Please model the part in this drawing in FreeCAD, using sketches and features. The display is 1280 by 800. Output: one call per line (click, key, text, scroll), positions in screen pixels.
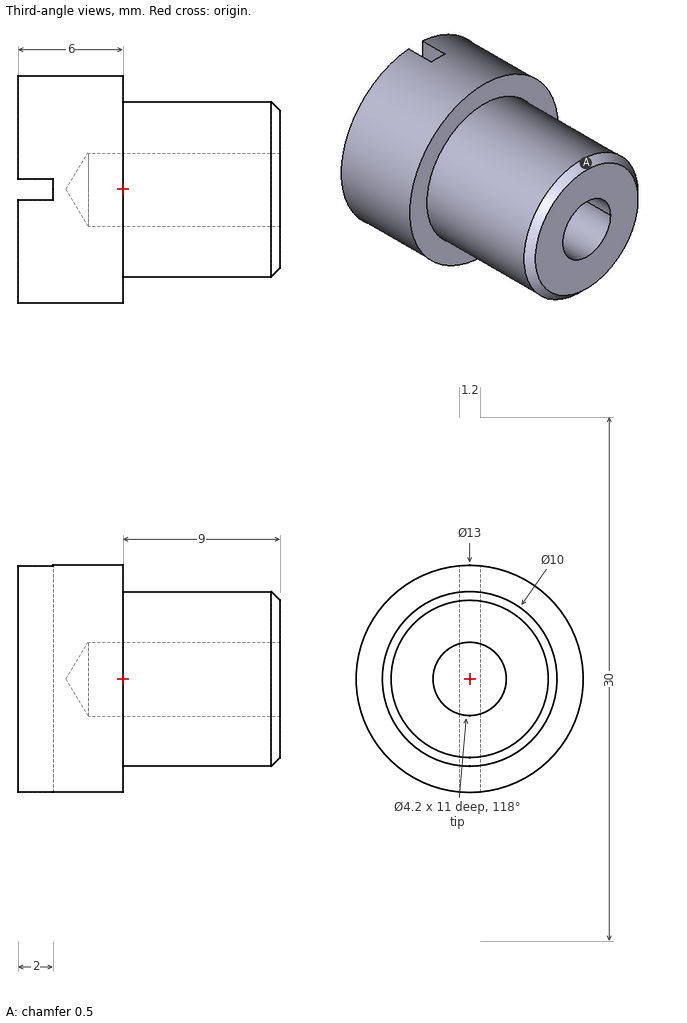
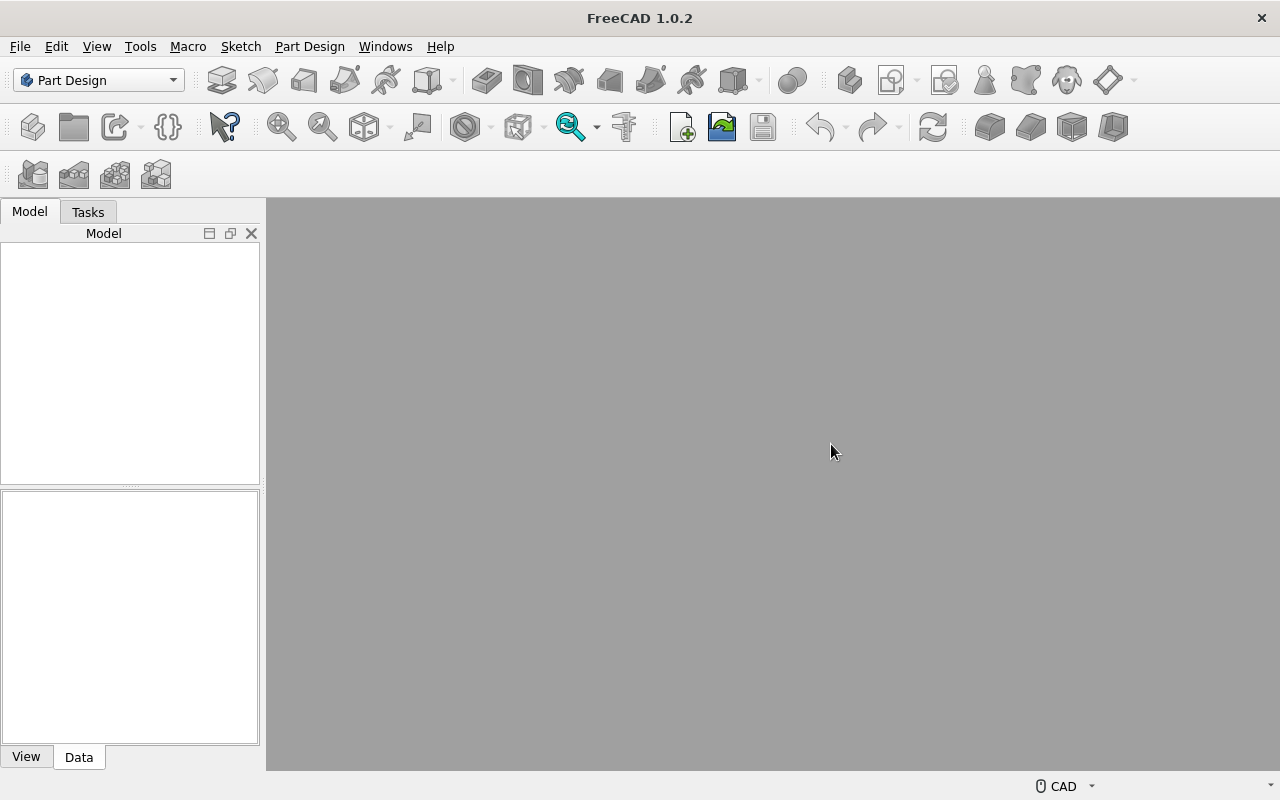
click(681, 128)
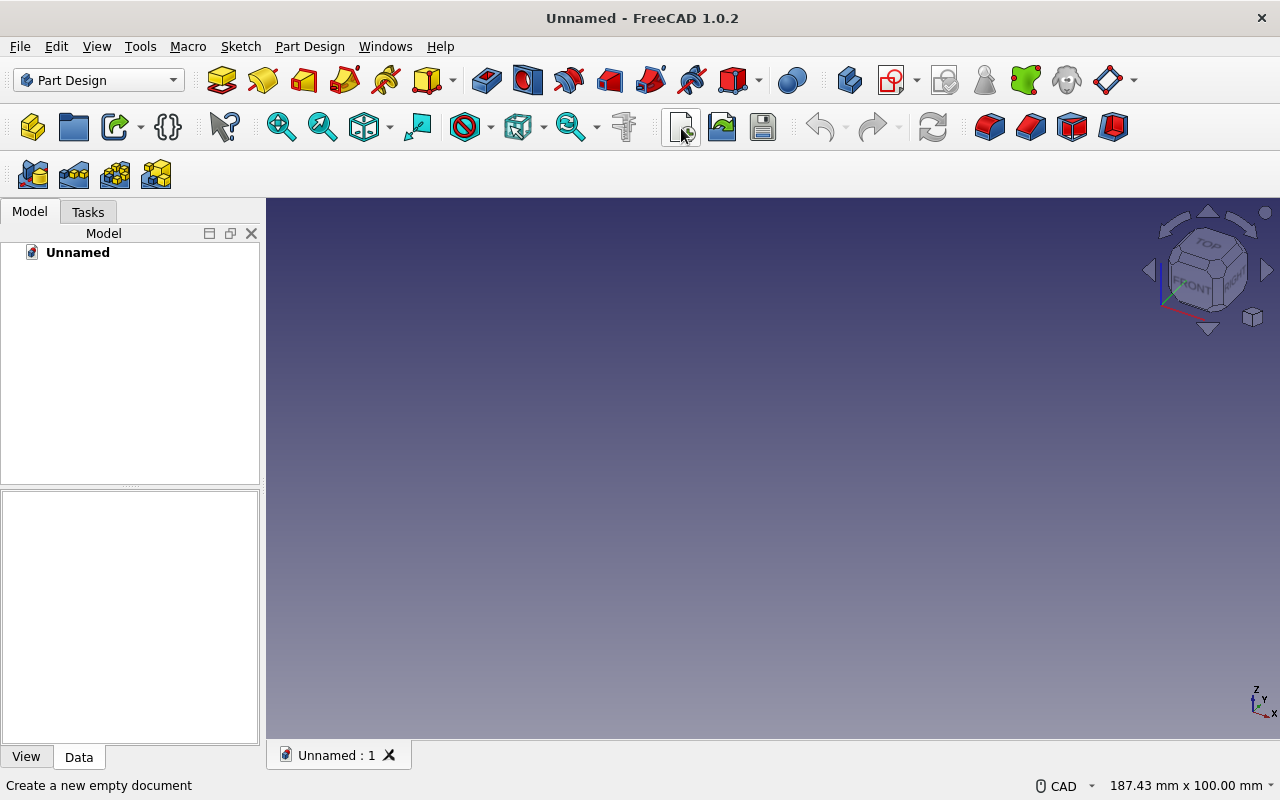
click(890, 80)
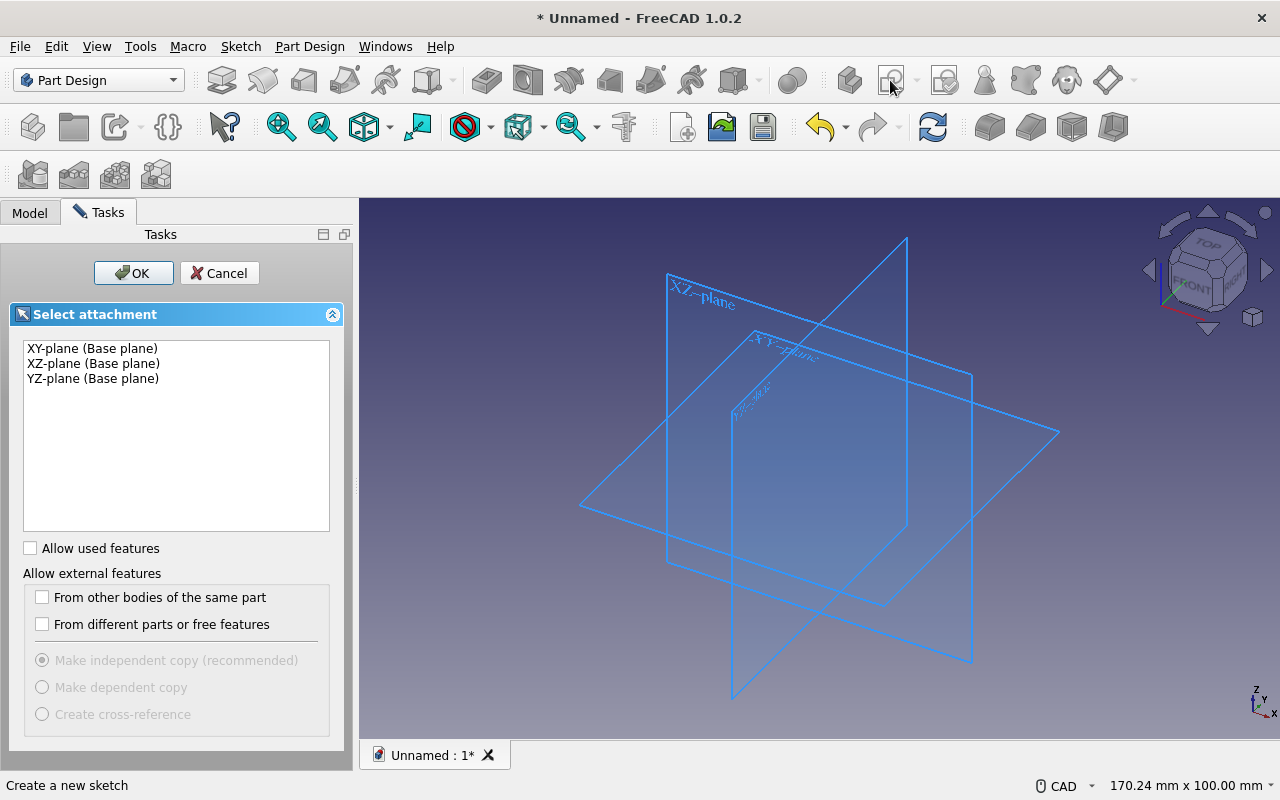
click(84, 378)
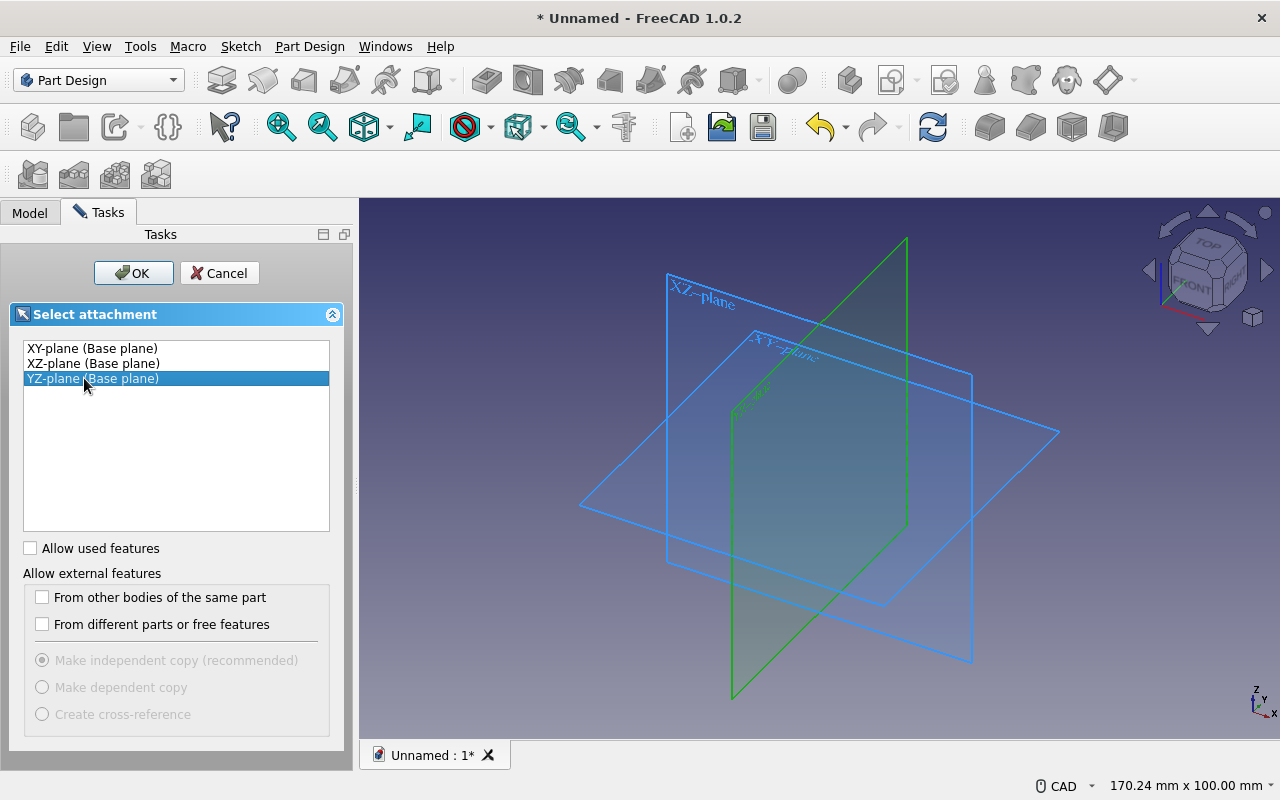
click(134, 273)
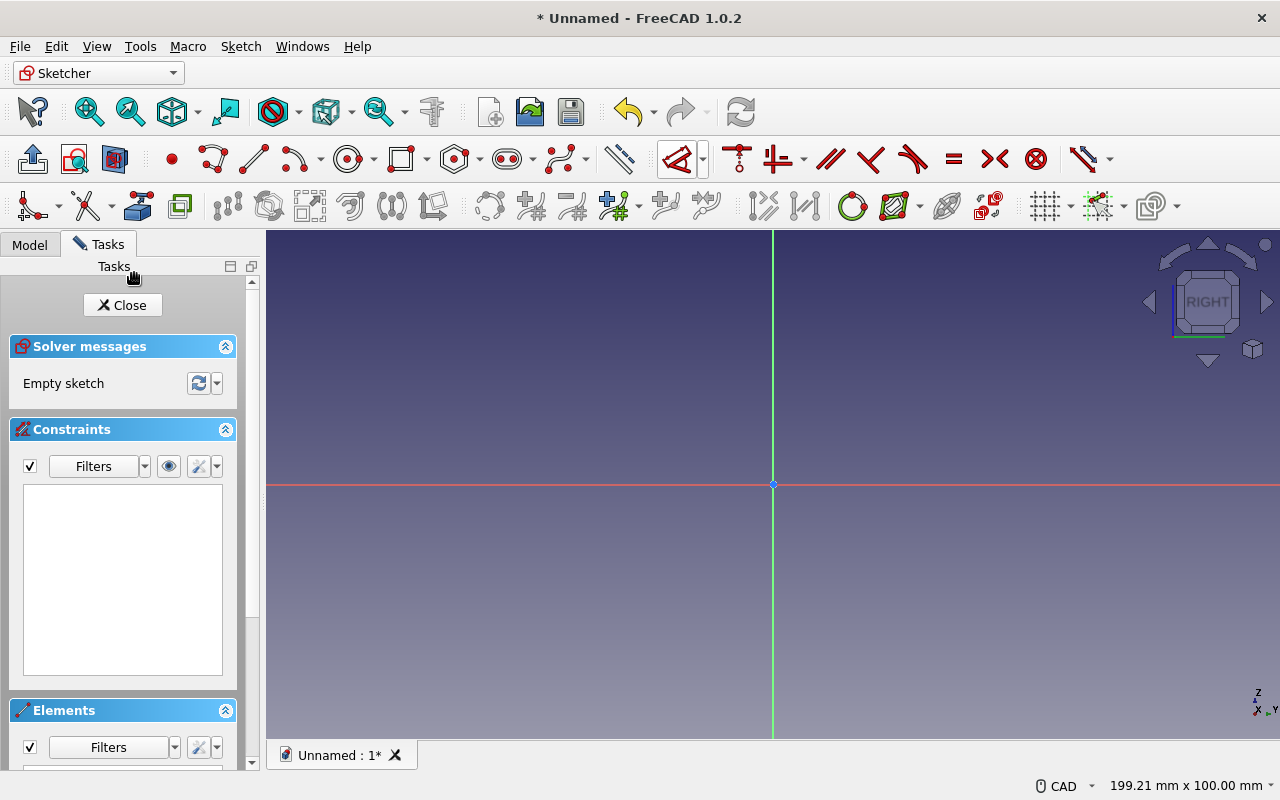
scroll(787, 484, up, 9)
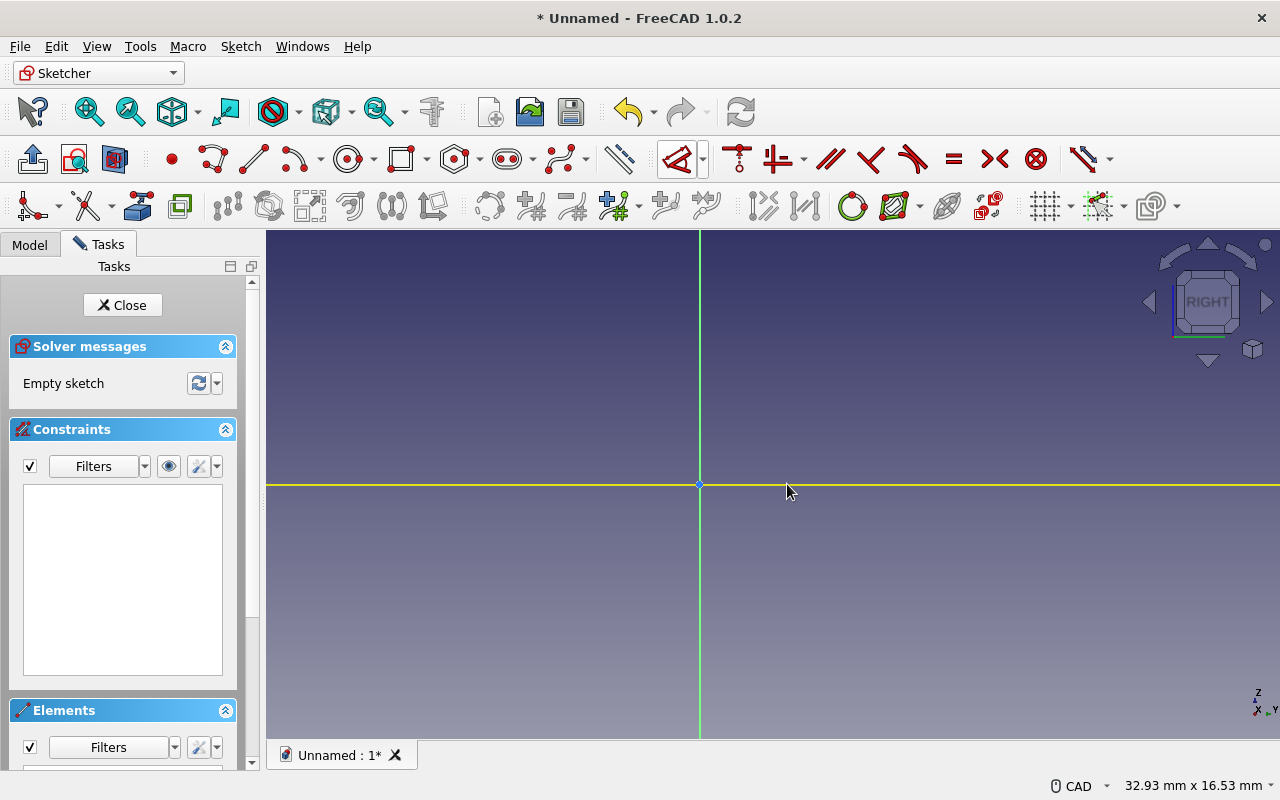
click(348, 160)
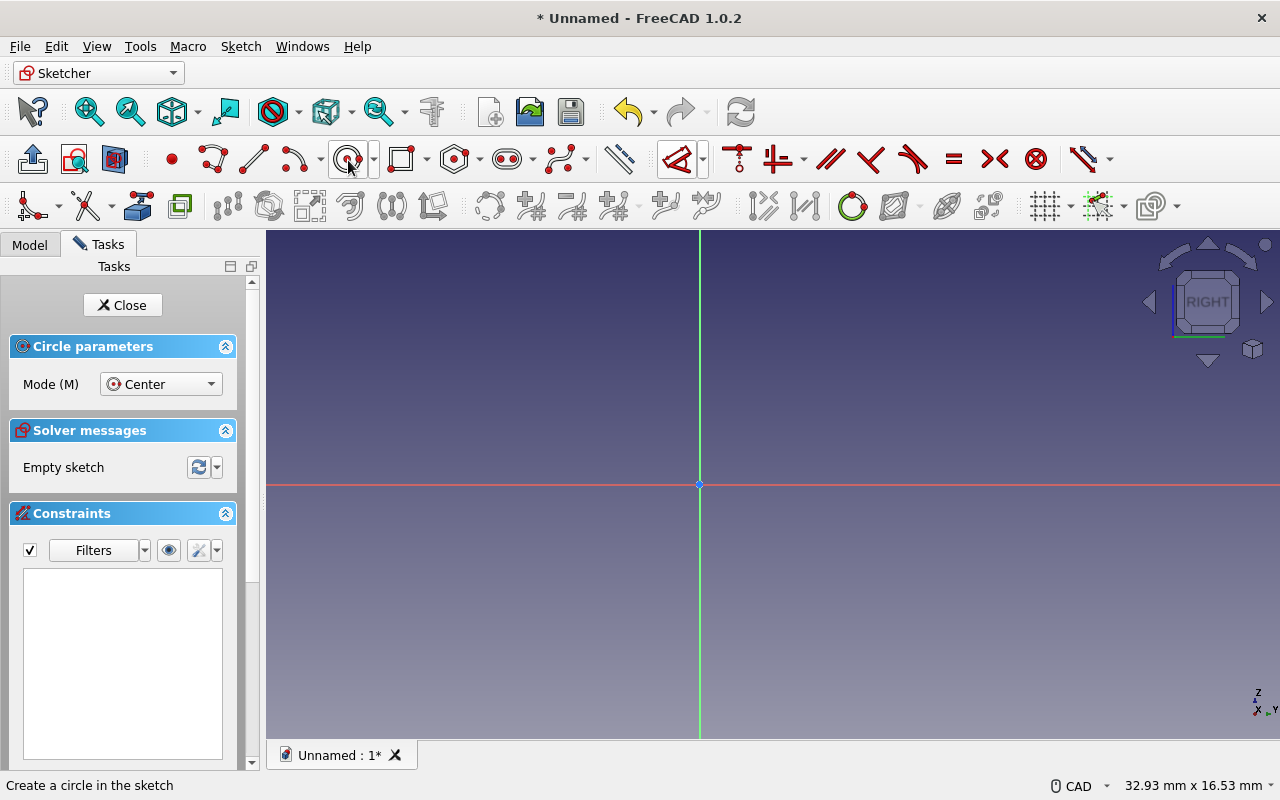
click(700, 484)
move(809, 376)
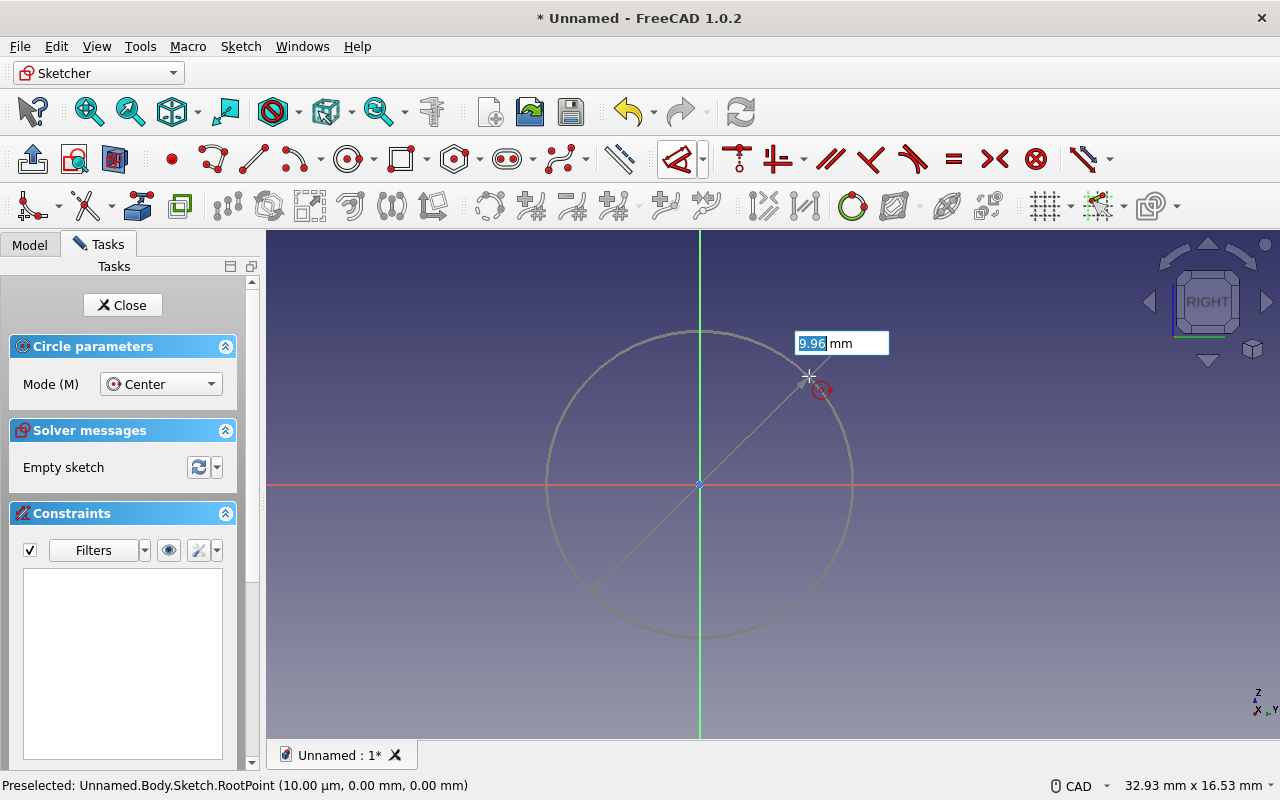
text(10)
key(Return)
key(Escape)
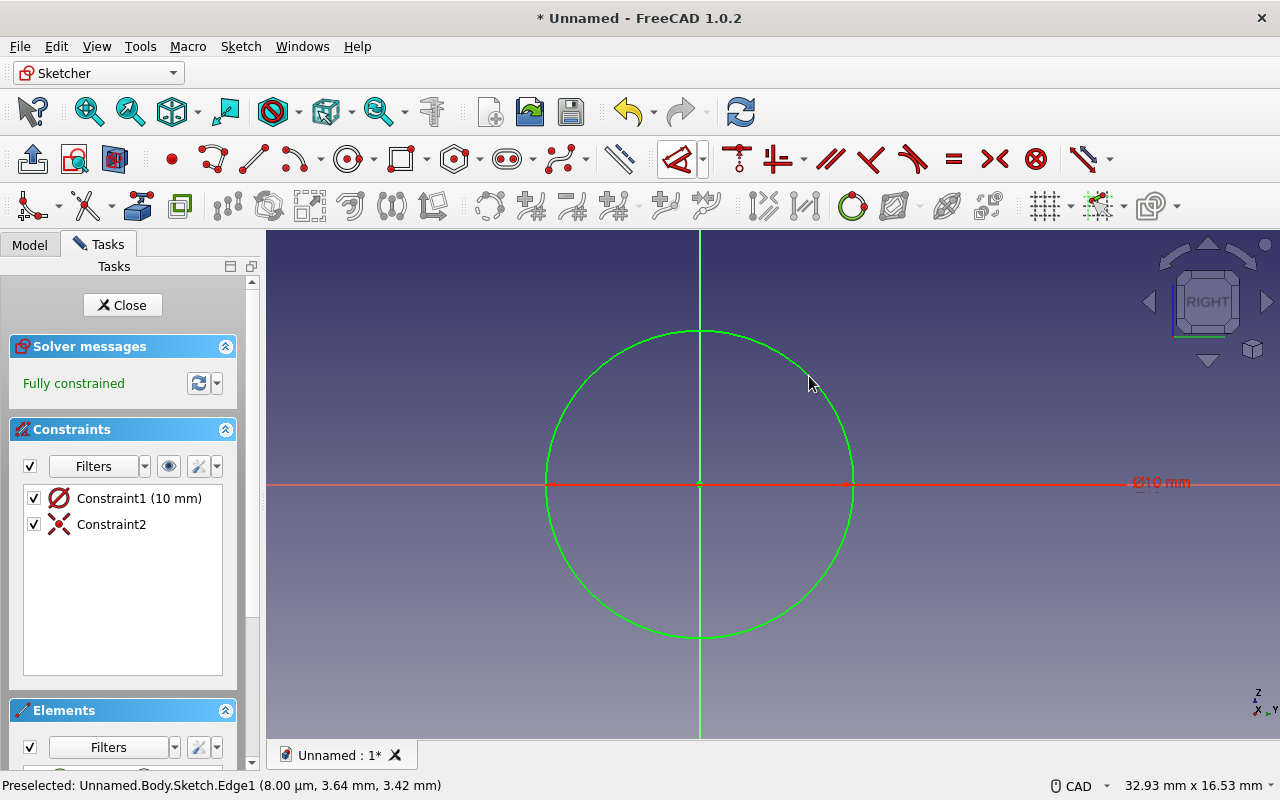
click(123, 305)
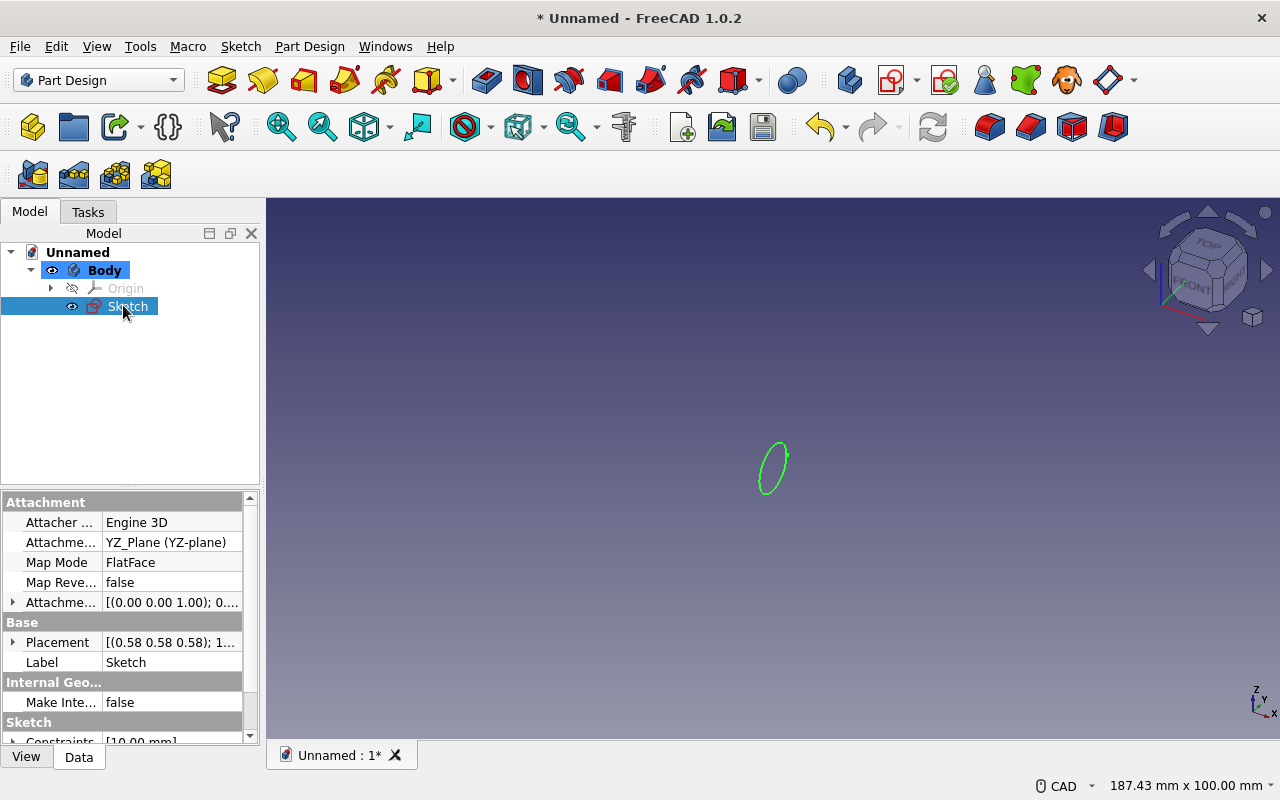
click(222, 80)